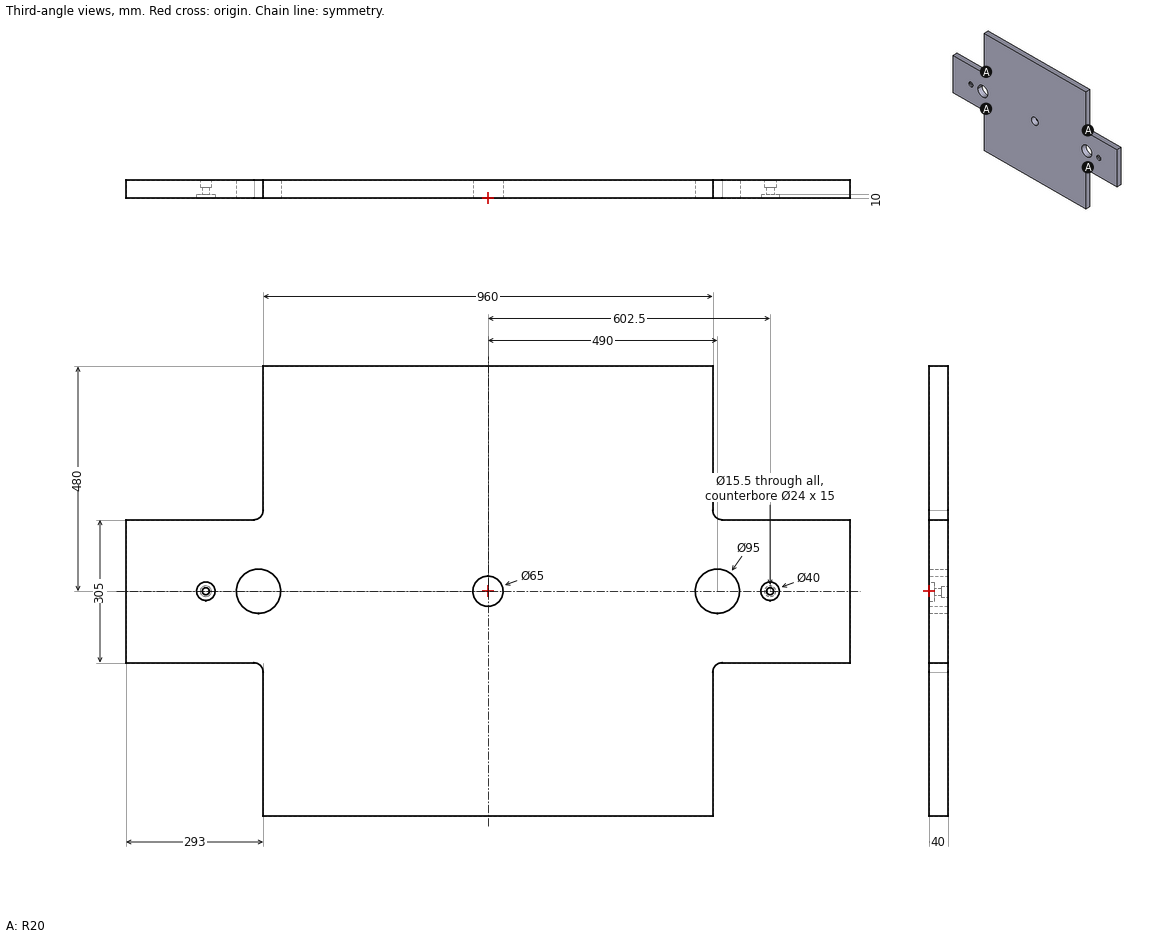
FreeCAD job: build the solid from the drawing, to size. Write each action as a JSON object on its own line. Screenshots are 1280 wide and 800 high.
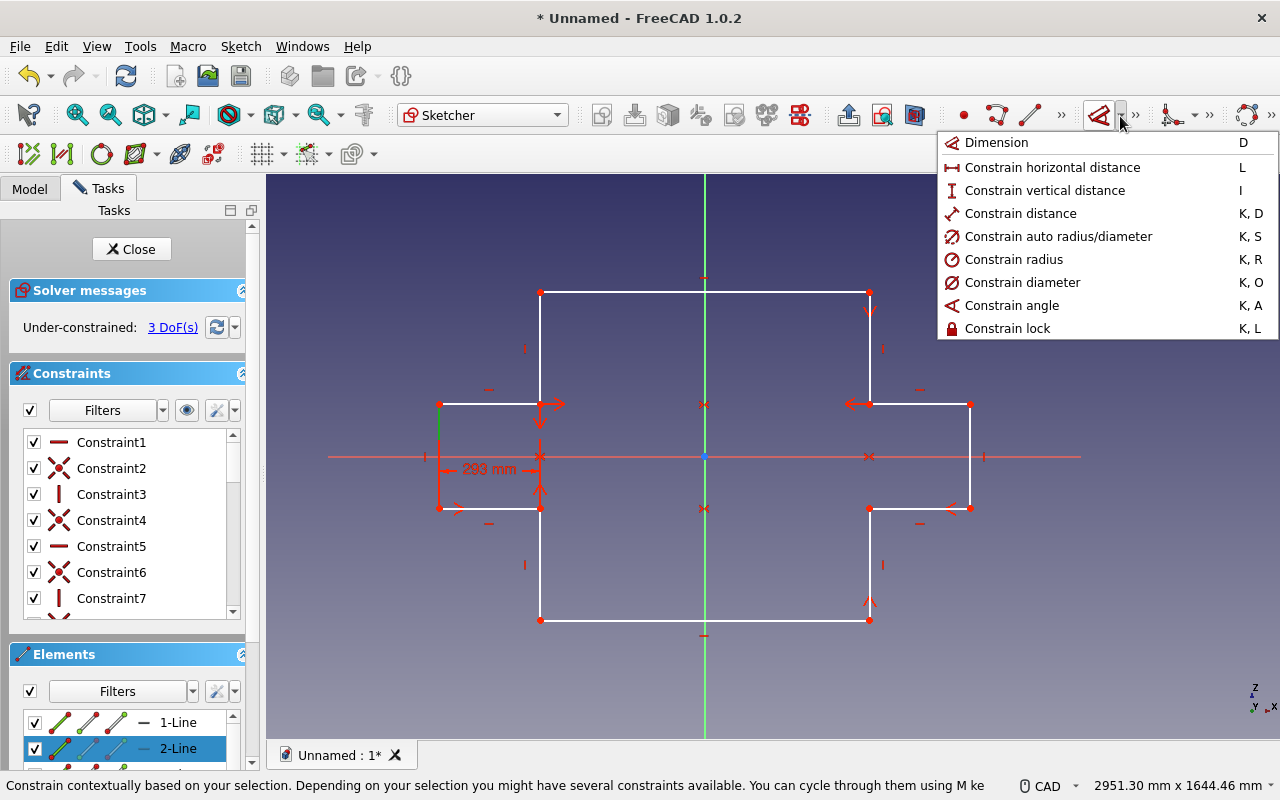
{"action": "left_click", "coordinate": [1108, 190]}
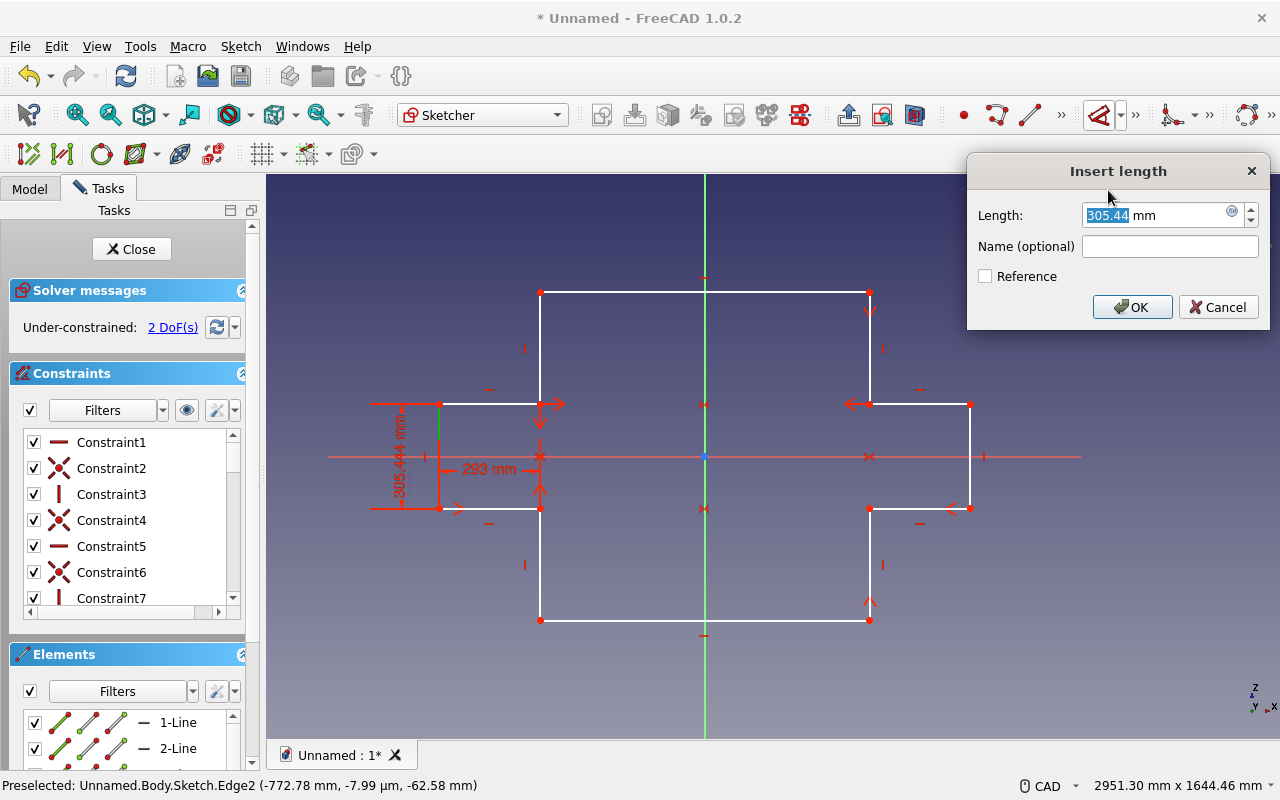
{"action": "type", "text": "305"}
{"action": "key", "text": "Return"}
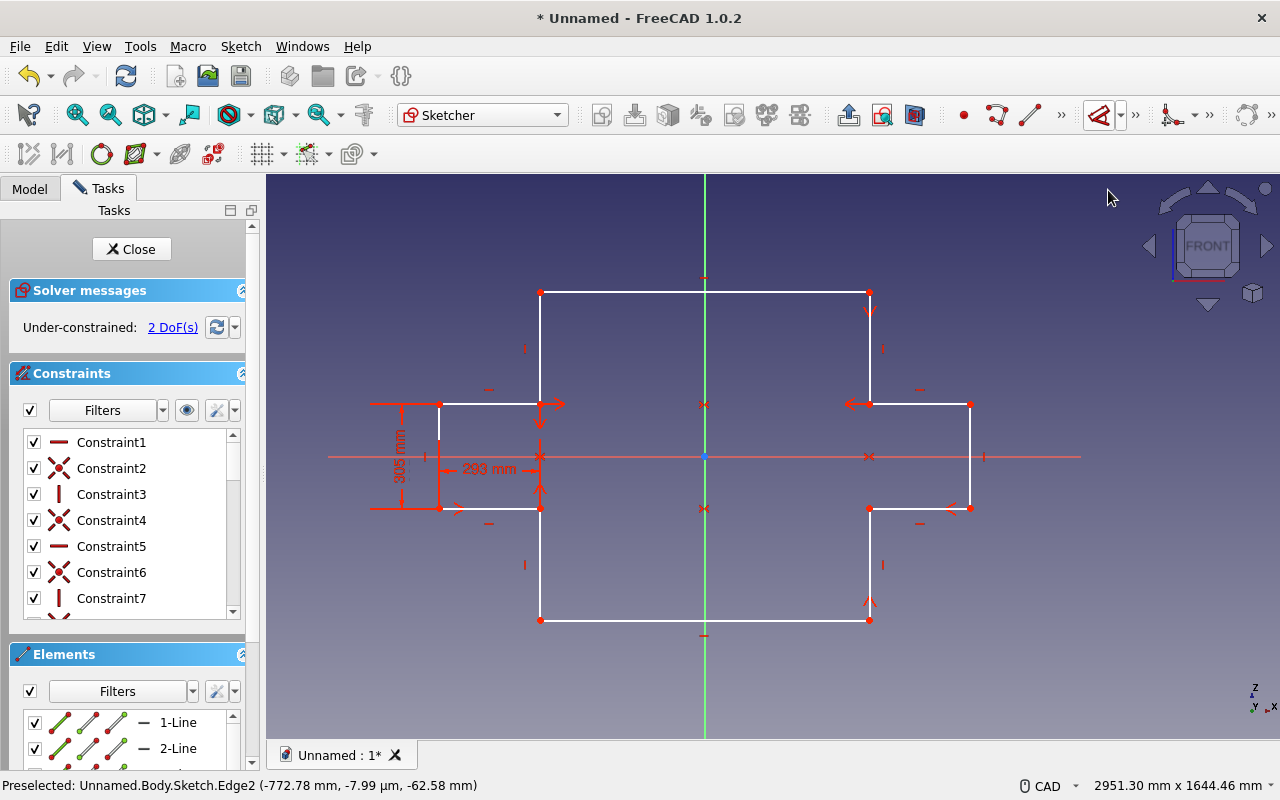
{"action": "left_click", "coordinate": [639, 292]}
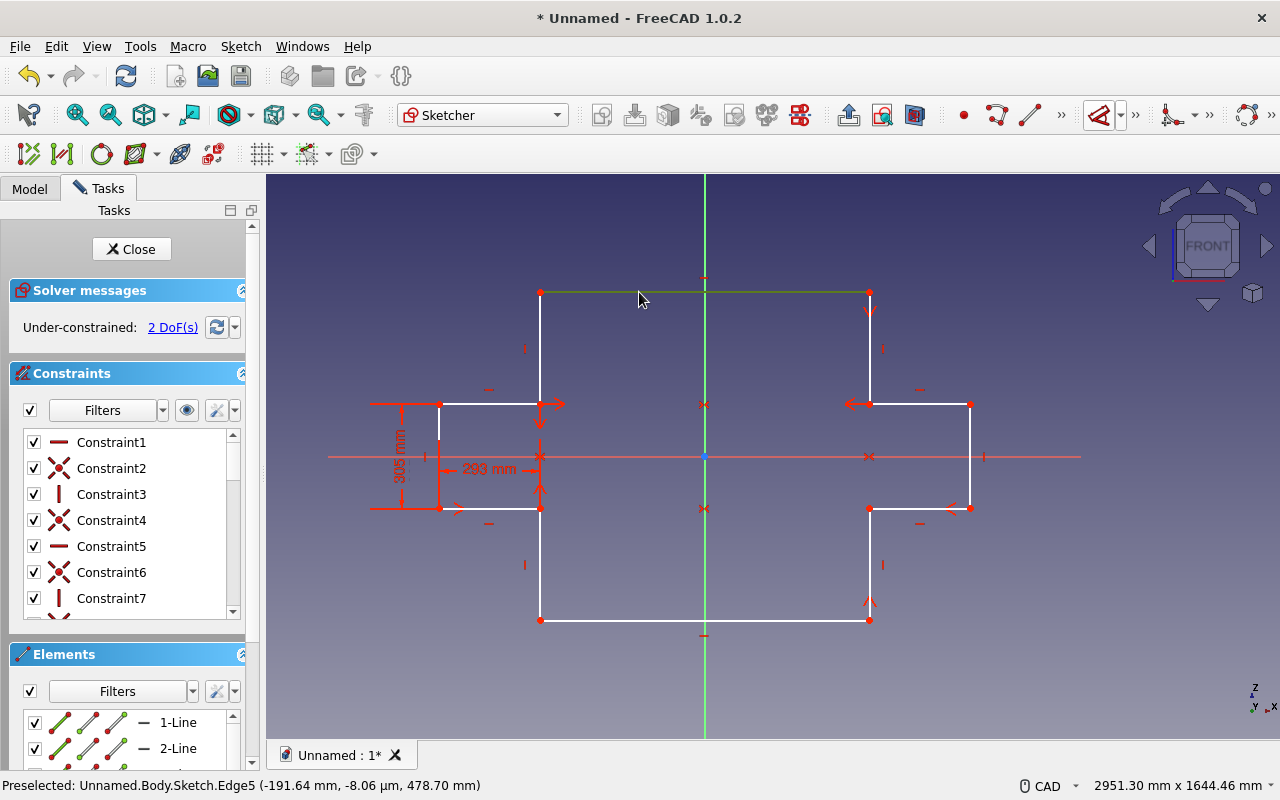
{"action": "key", "text": "l"}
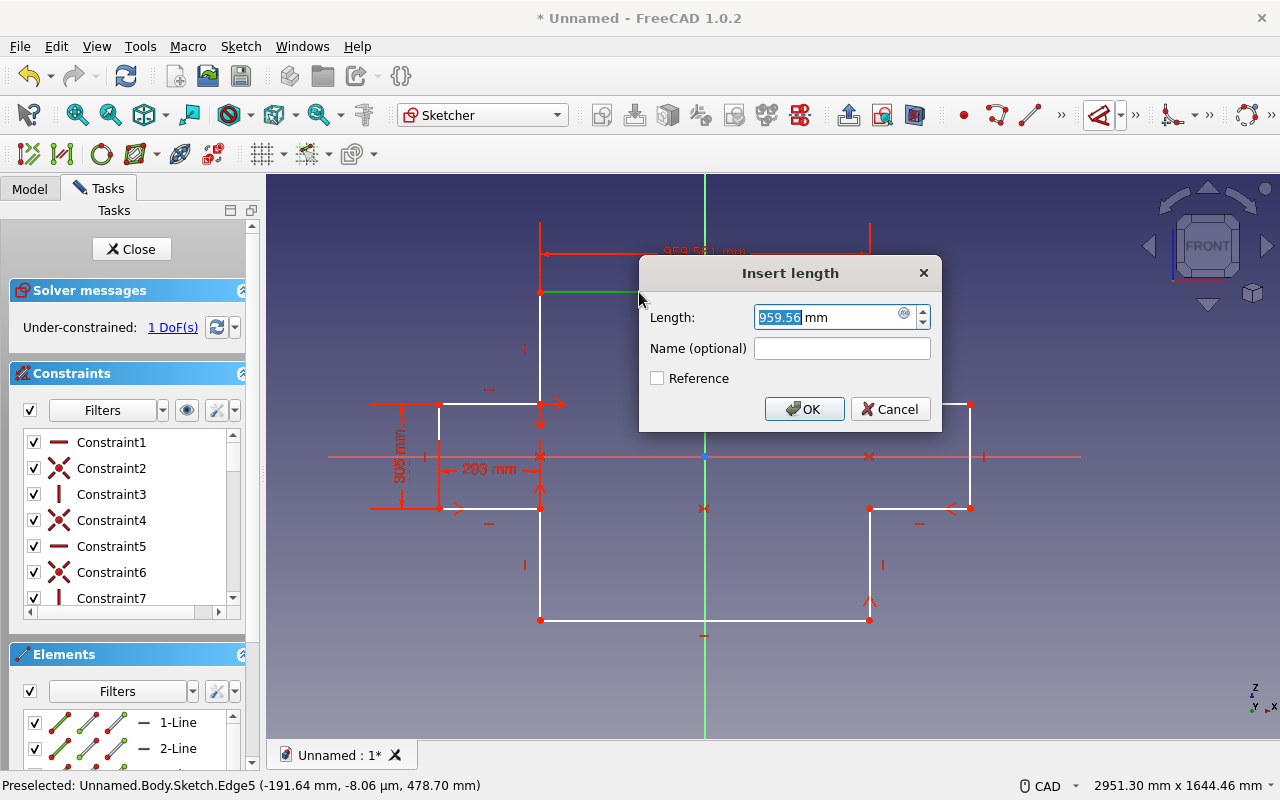
{"action": "type", "text": "960"}
{"action": "key", "text": "Return"}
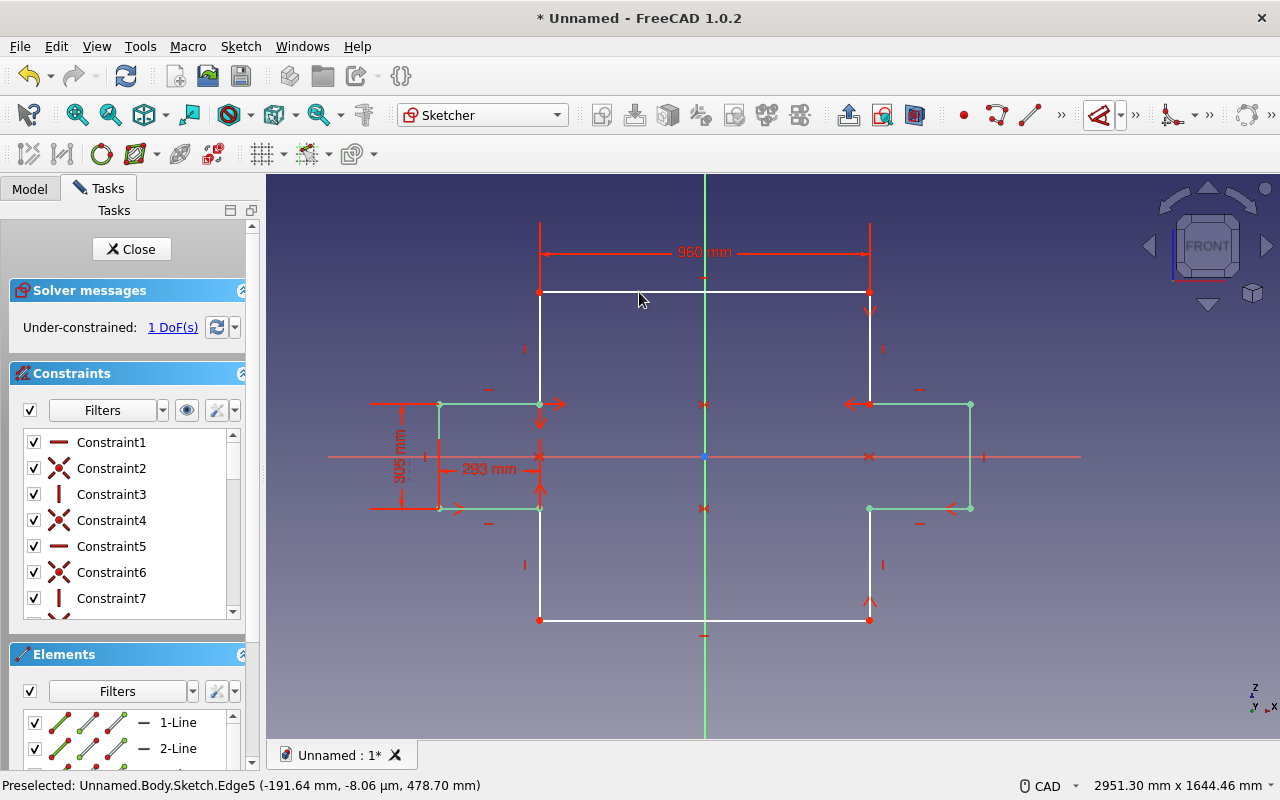
{"action": "left_click", "coordinate": [540, 292]}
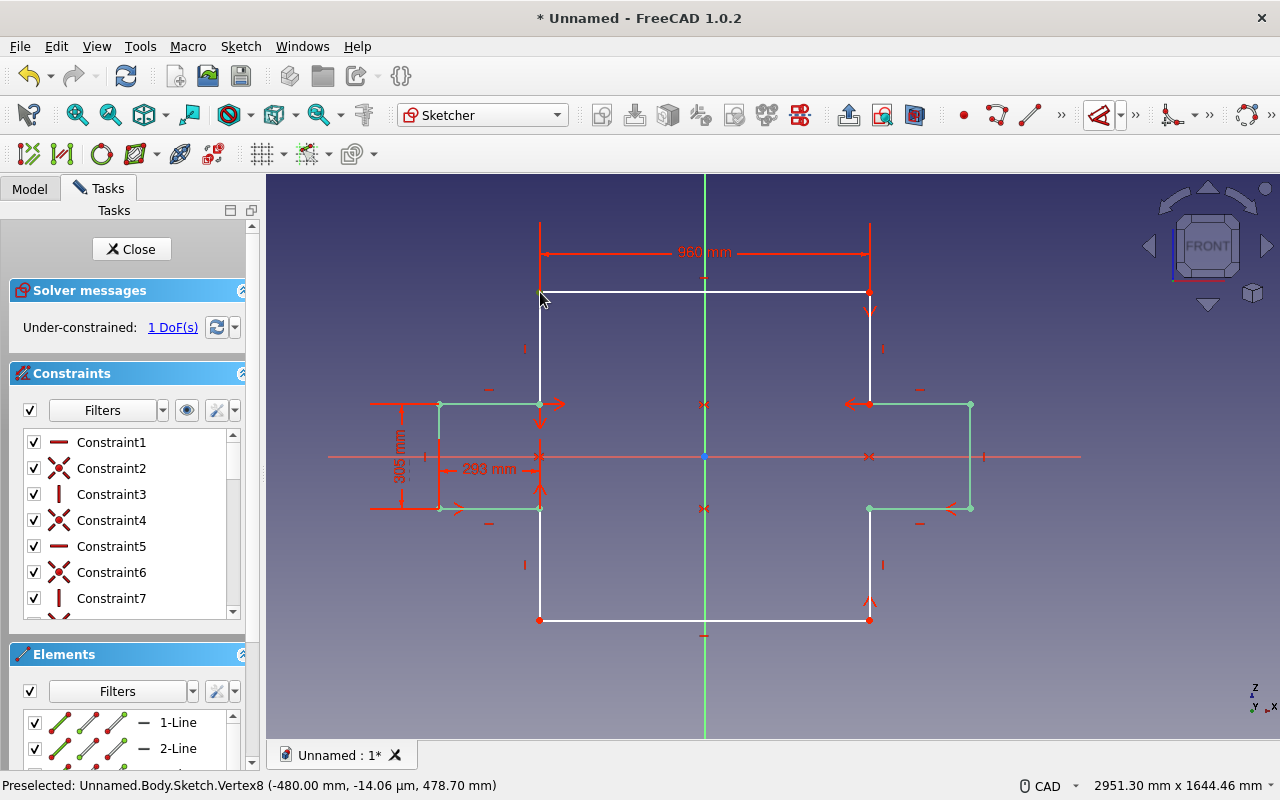
{"action": "left_click", "coordinate": [1120, 116]}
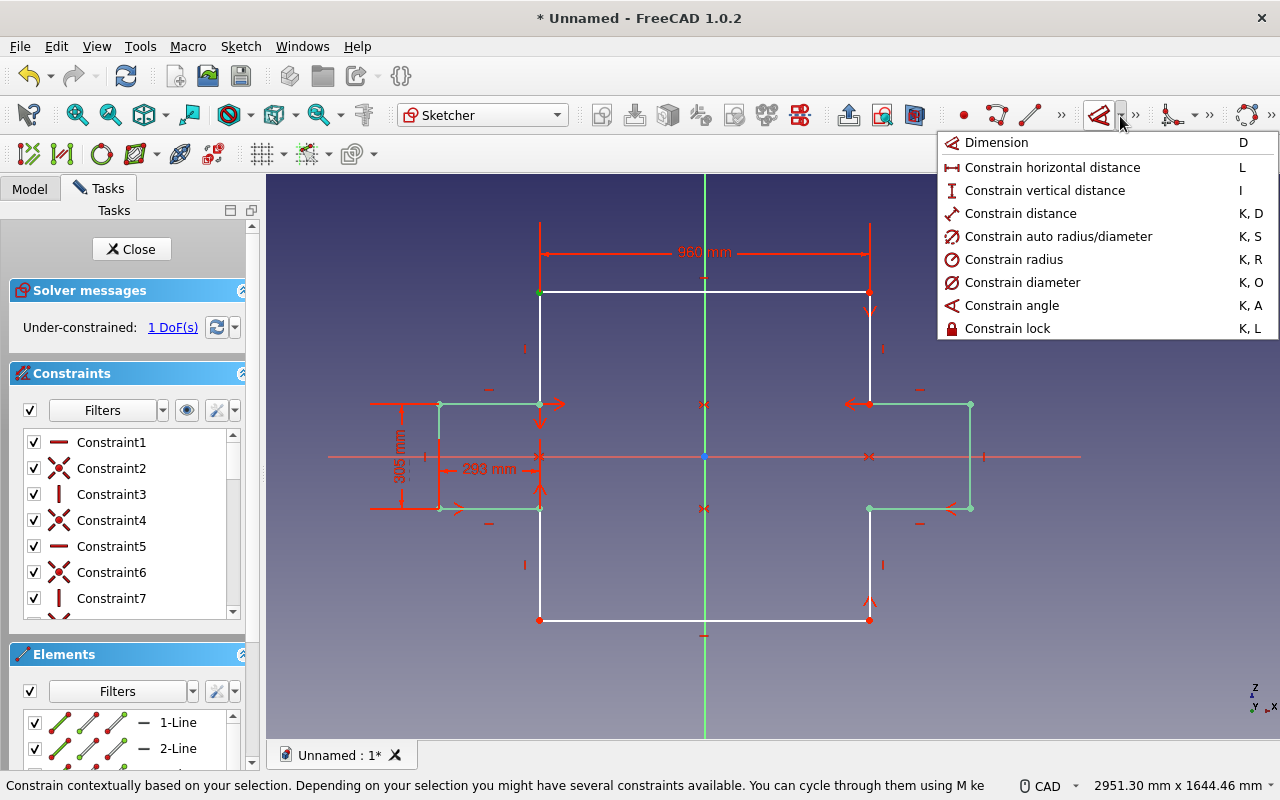
{"action": "left_click", "coordinate": [1108, 190]}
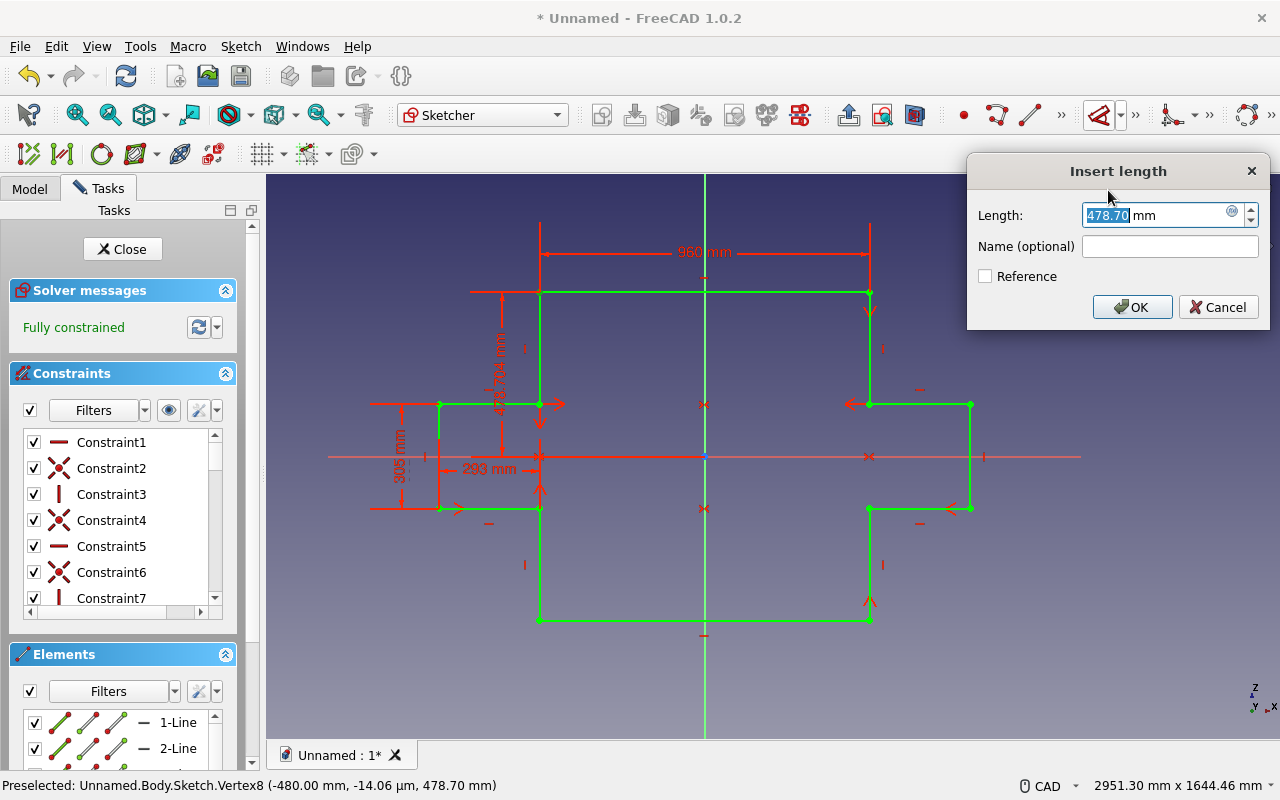
{"action": "type", "text": "480"}
{"action": "key", "text": "Return"}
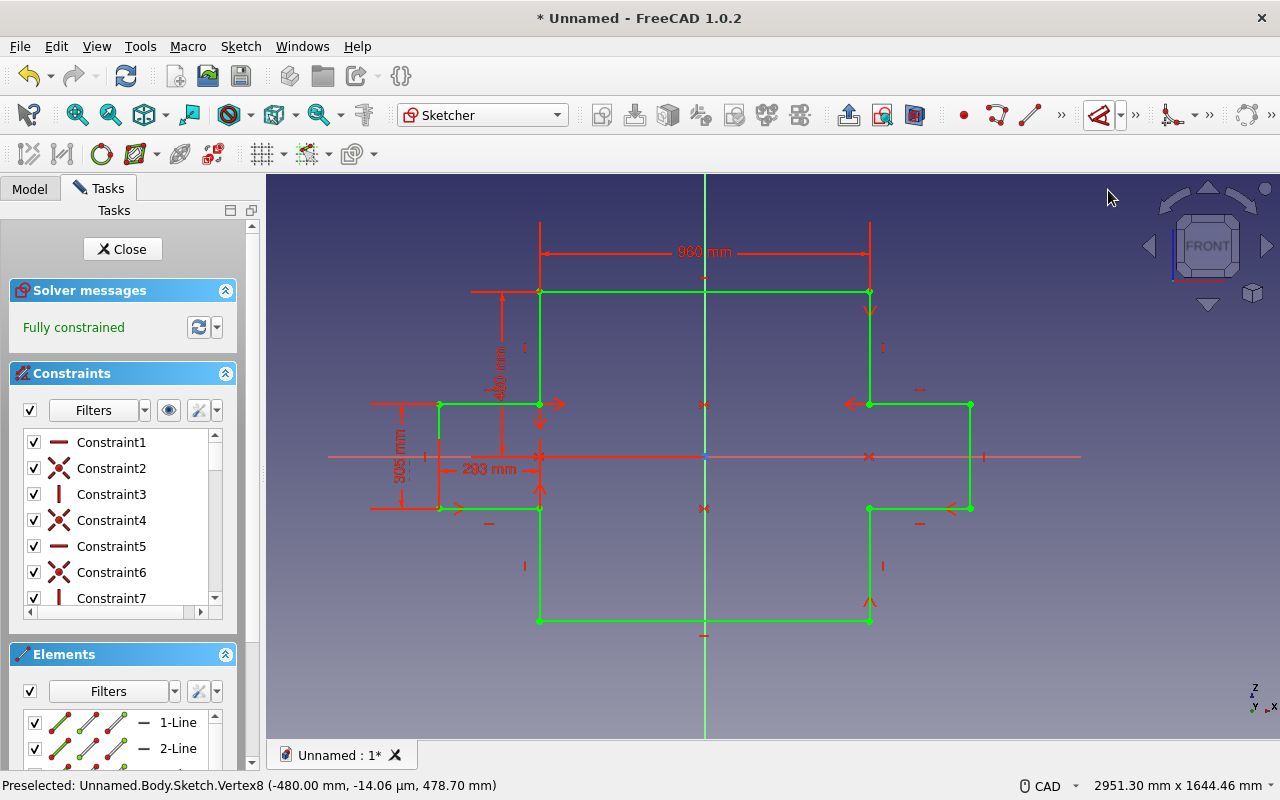
{"action": "left_click", "coordinate": [123, 249]}